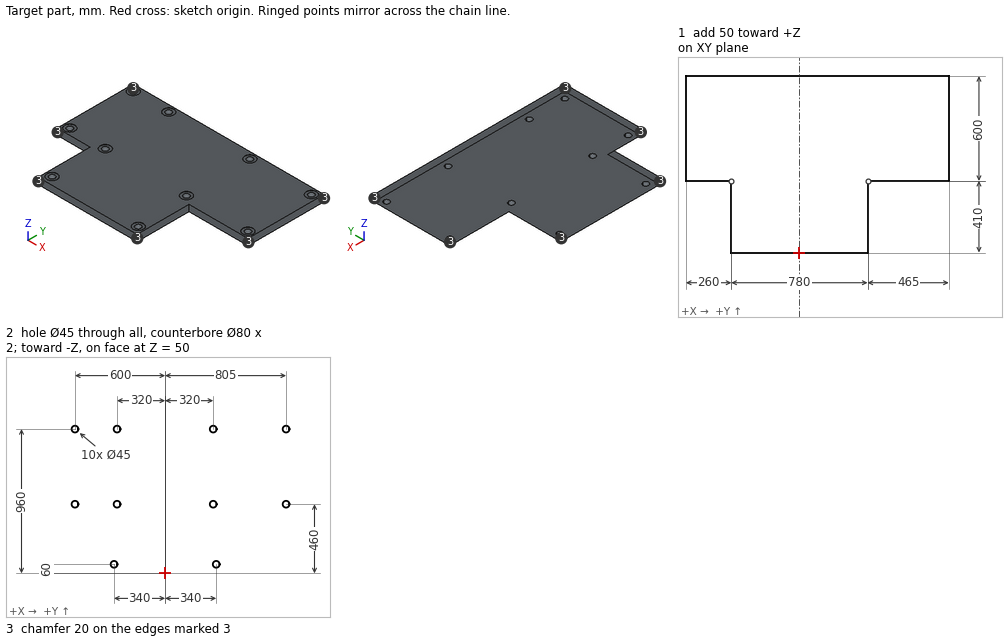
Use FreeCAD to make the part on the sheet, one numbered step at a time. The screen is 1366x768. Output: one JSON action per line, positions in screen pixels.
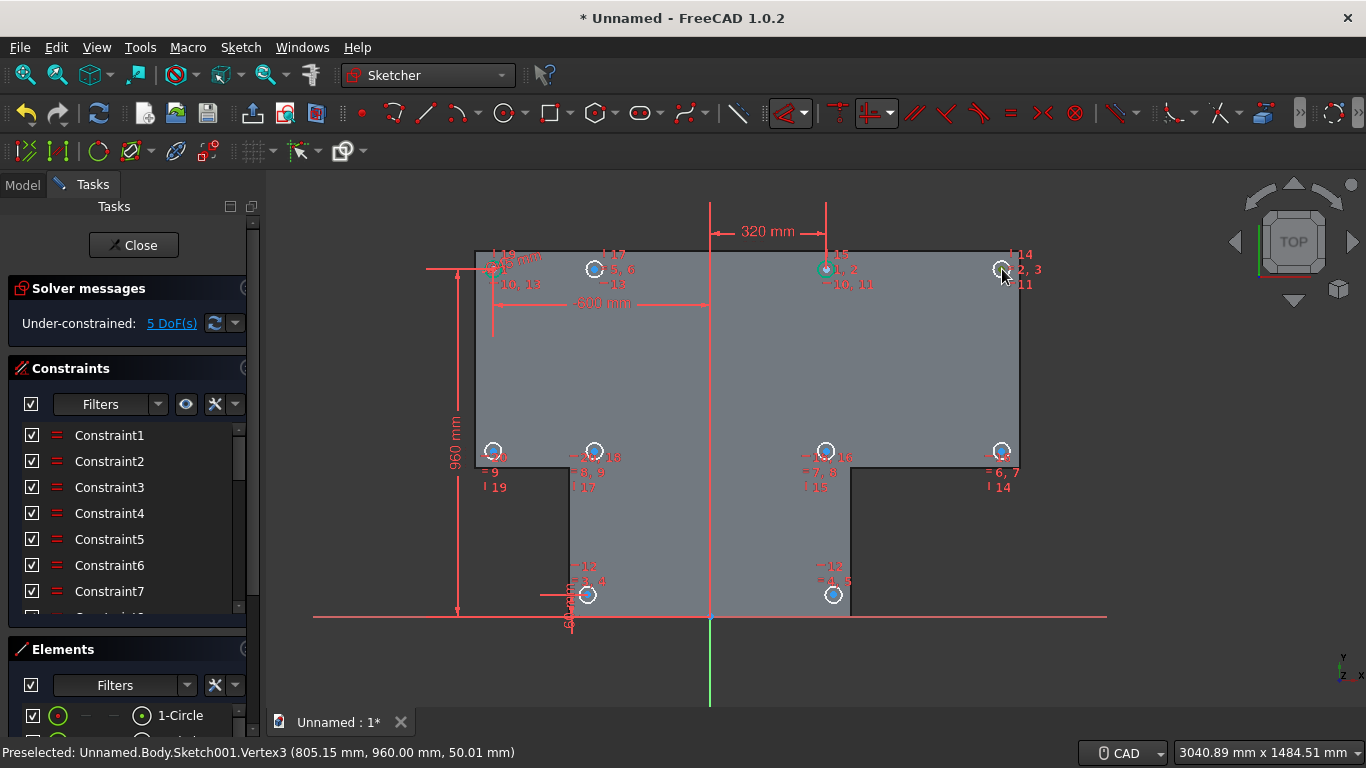
{"action": "key", "text": "l"}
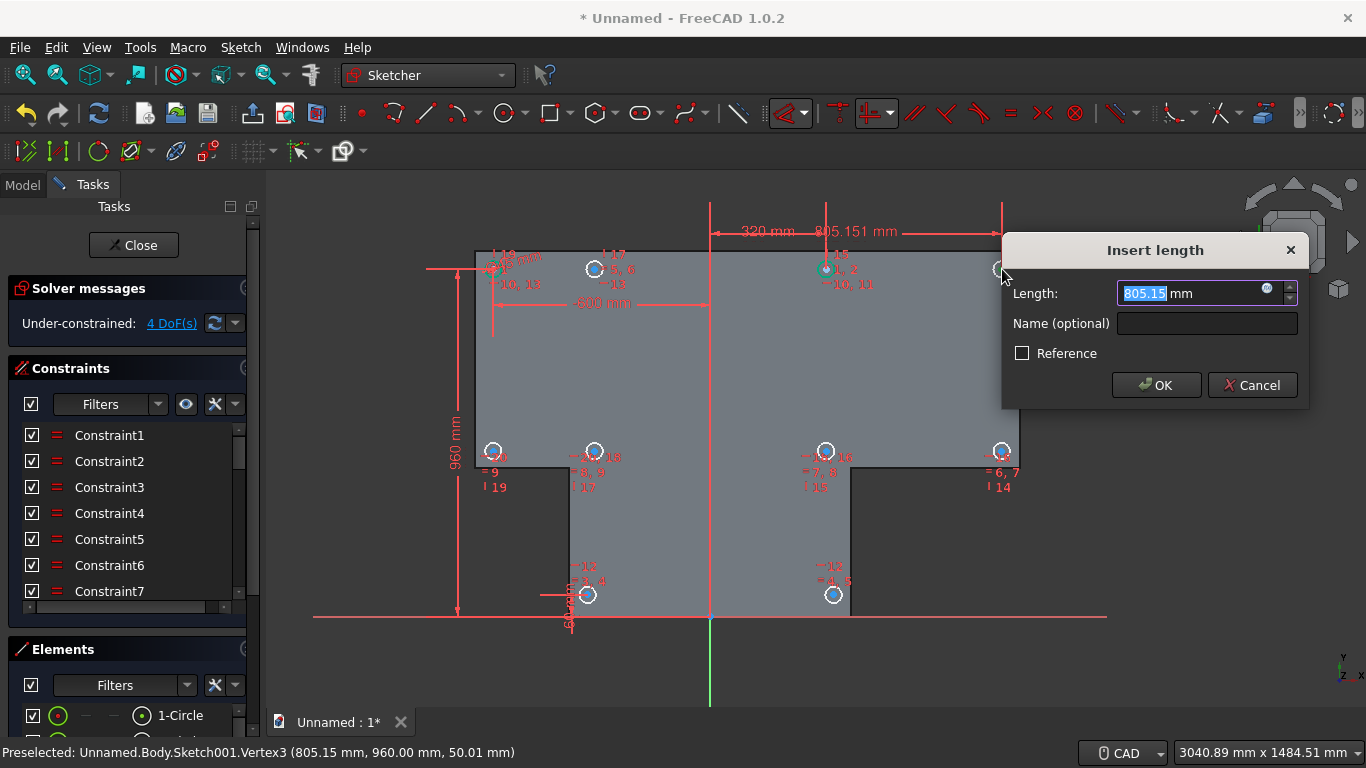
{"action": "type", "text": "805"}
{"action": "key", "text": "Return"}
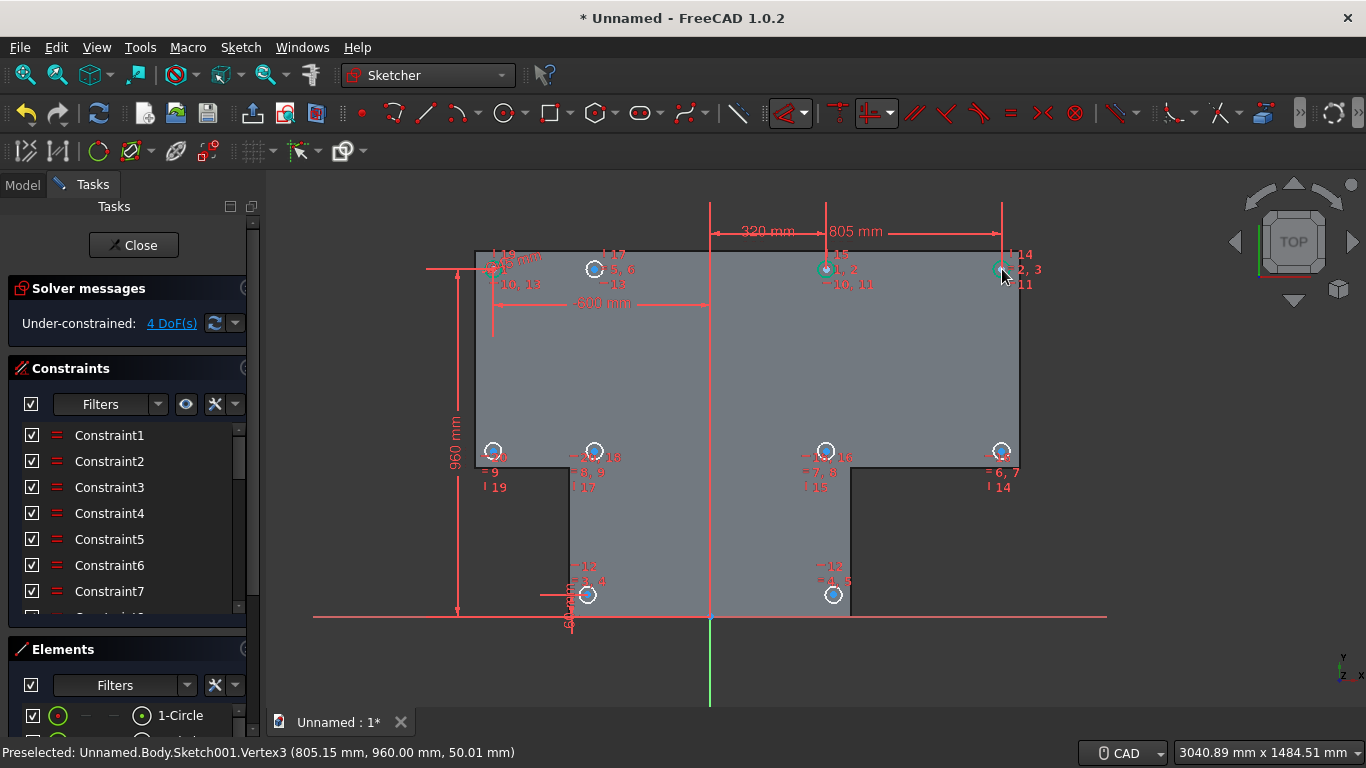
{"action": "left_click", "coordinate": [588, 595]}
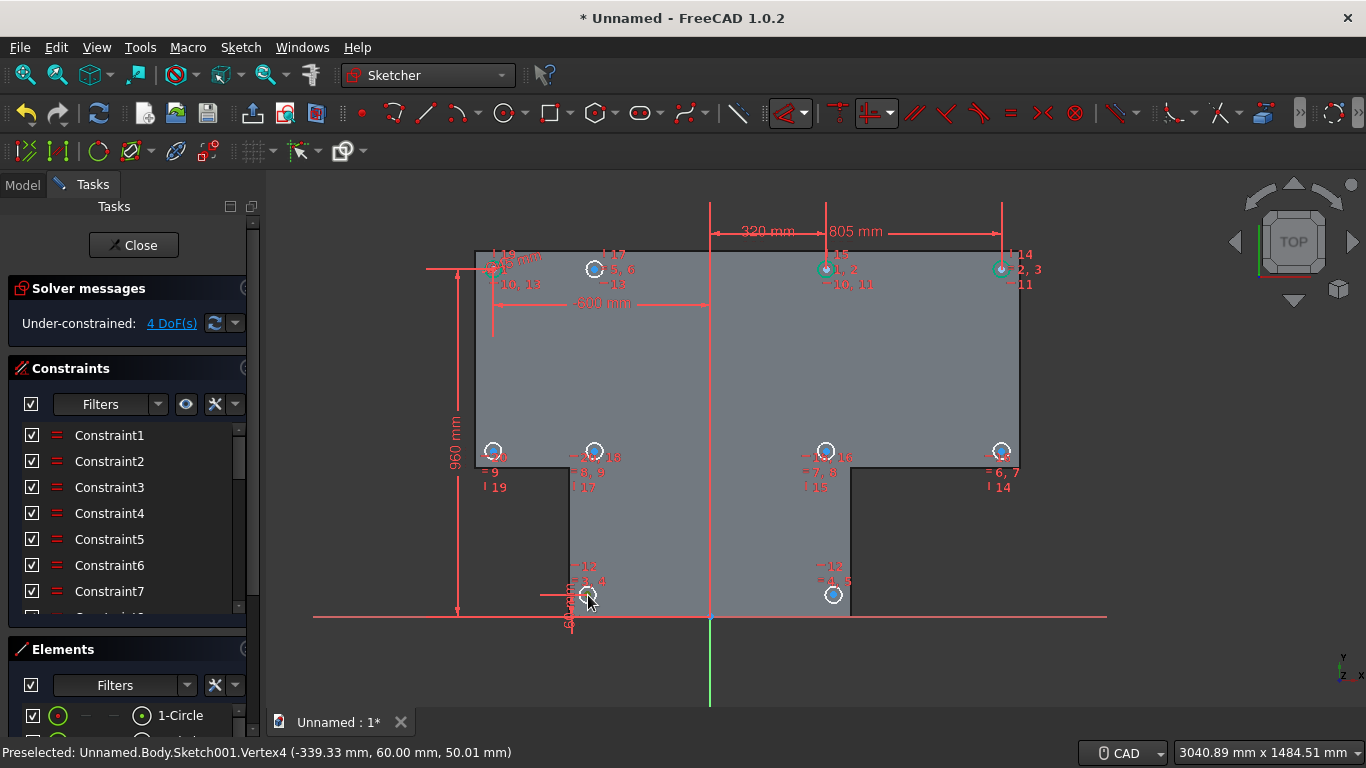
{"action": "left_click", "coordinate": [806, 114]}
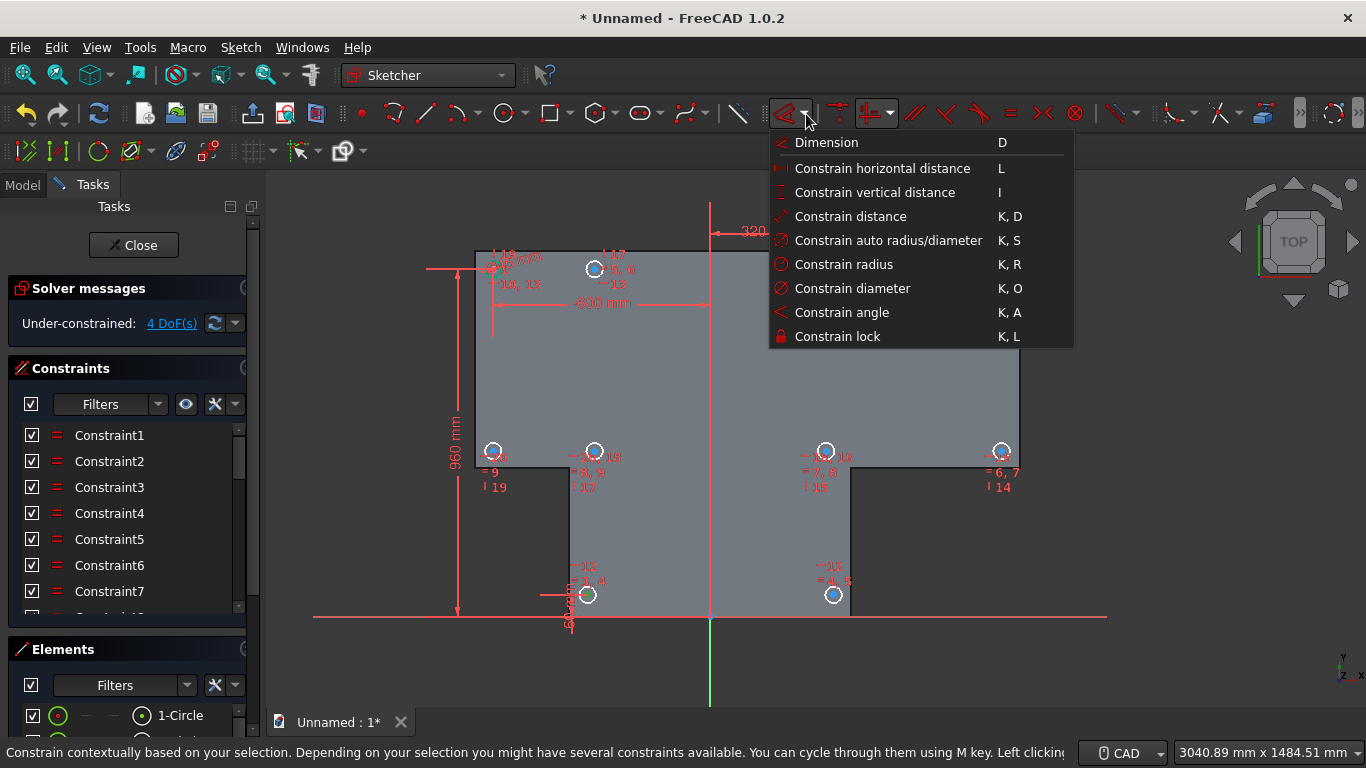
{"action": "left_click", "coordinate": [922, 168]}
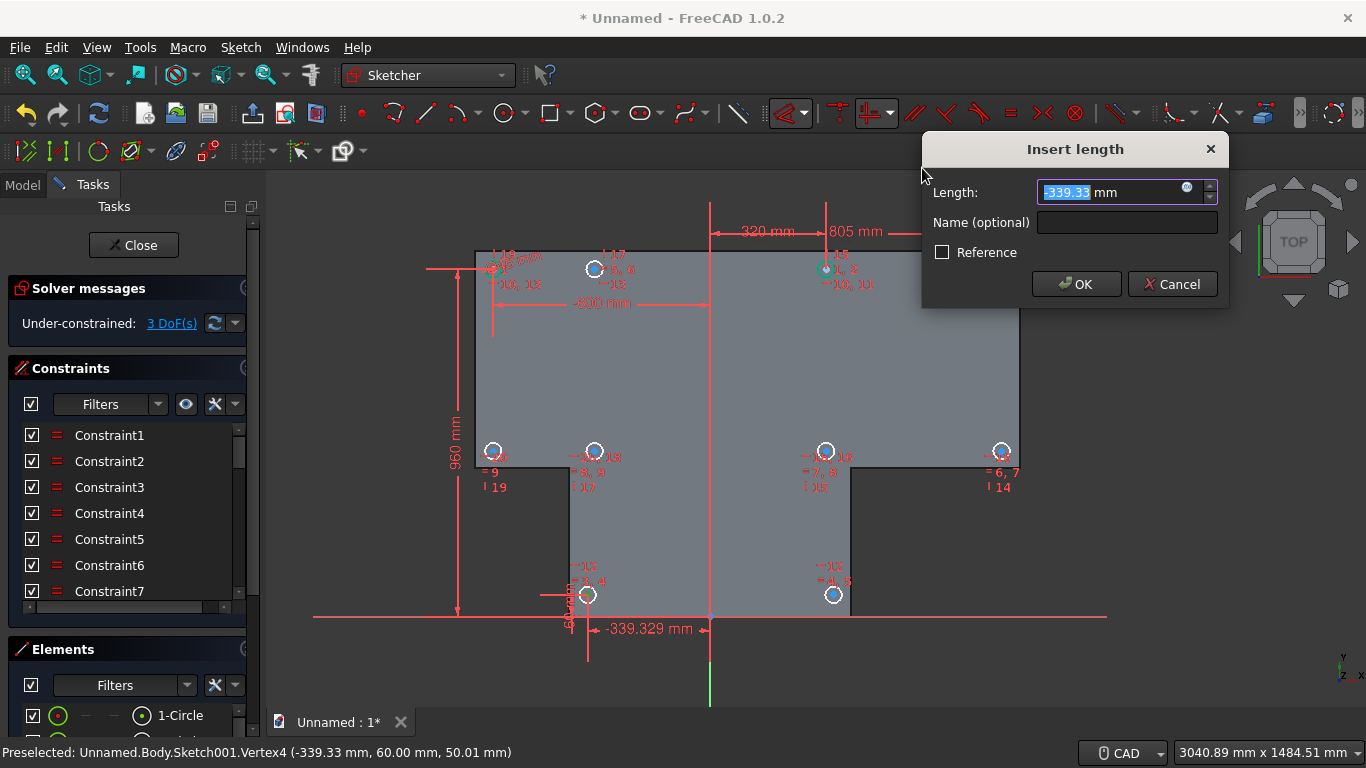
{"action": "type", "text": "-340"}
{"action": "key", "text": "Return"}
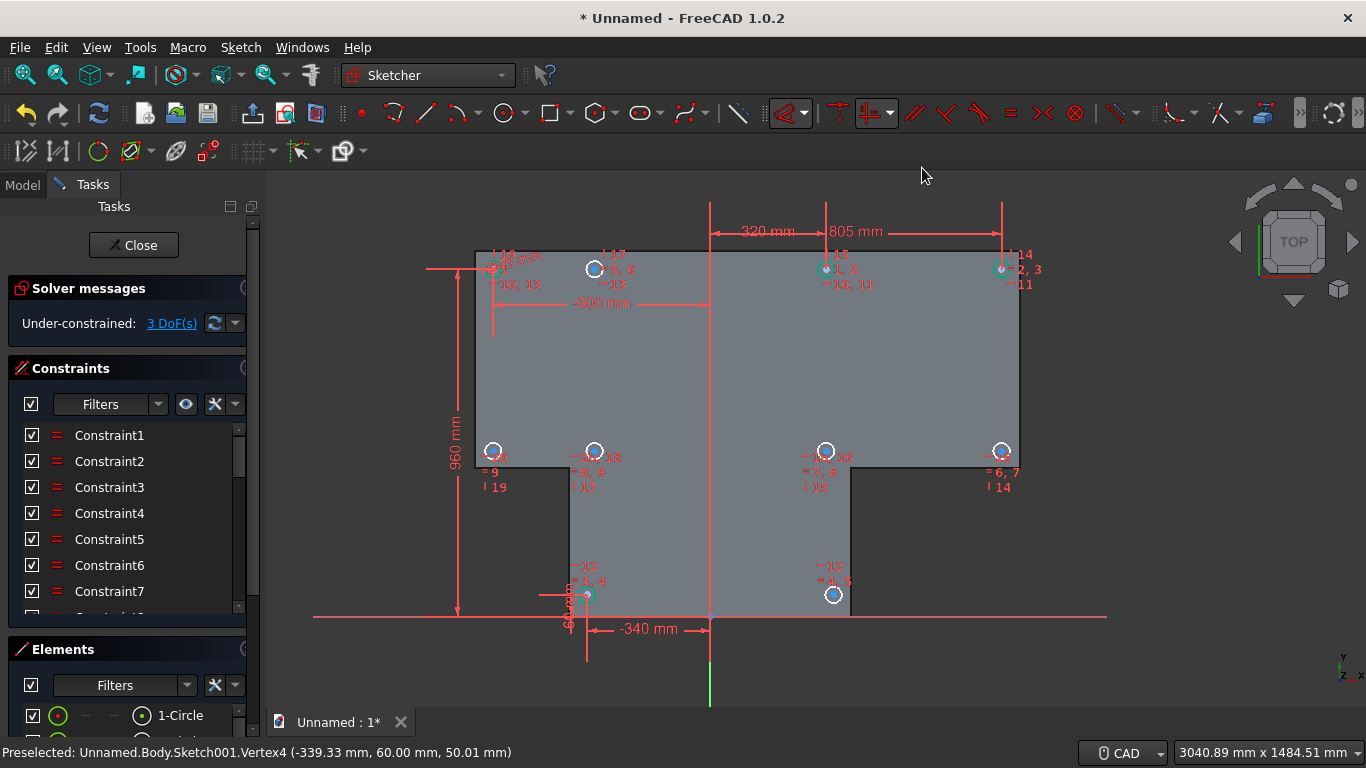
{"action": "left_click", "coordinate": [834, 595]}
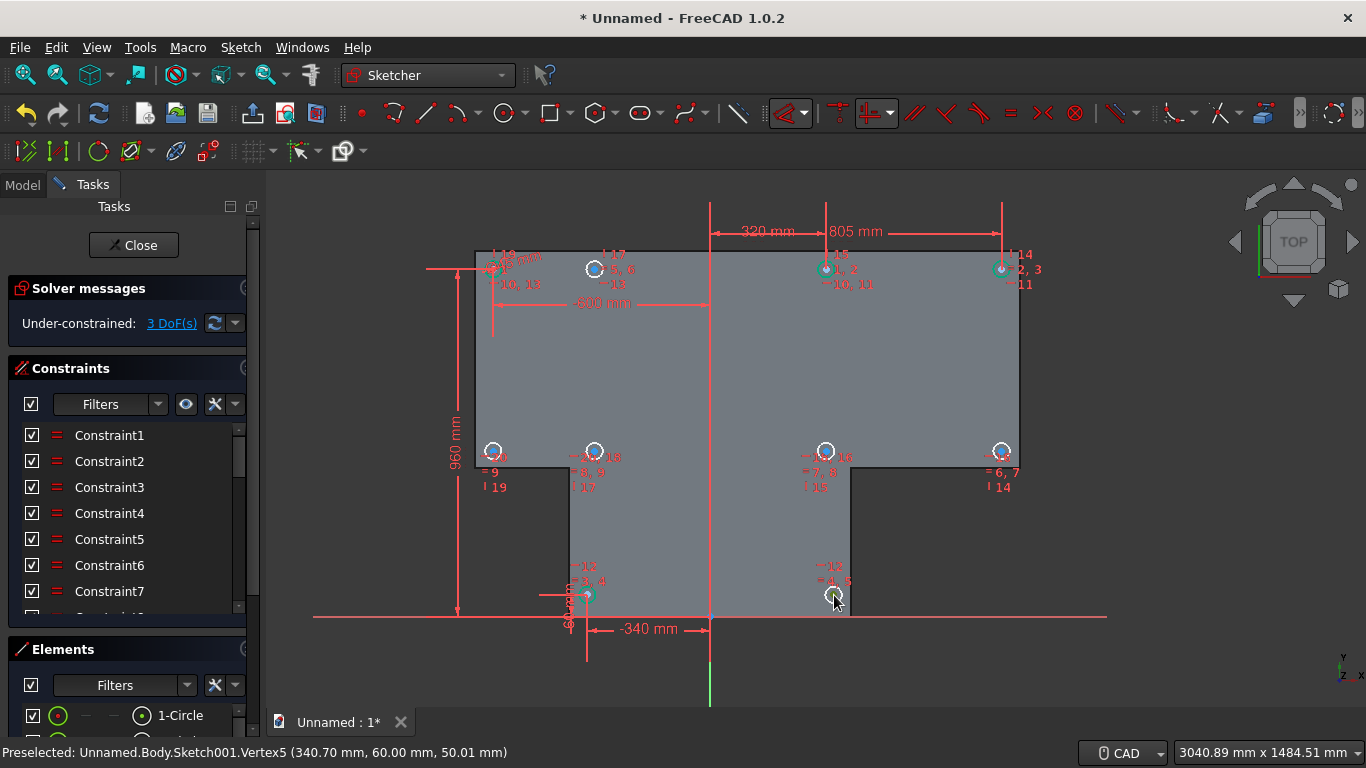
{"action": "left_click", "coordinate": [806, 114]}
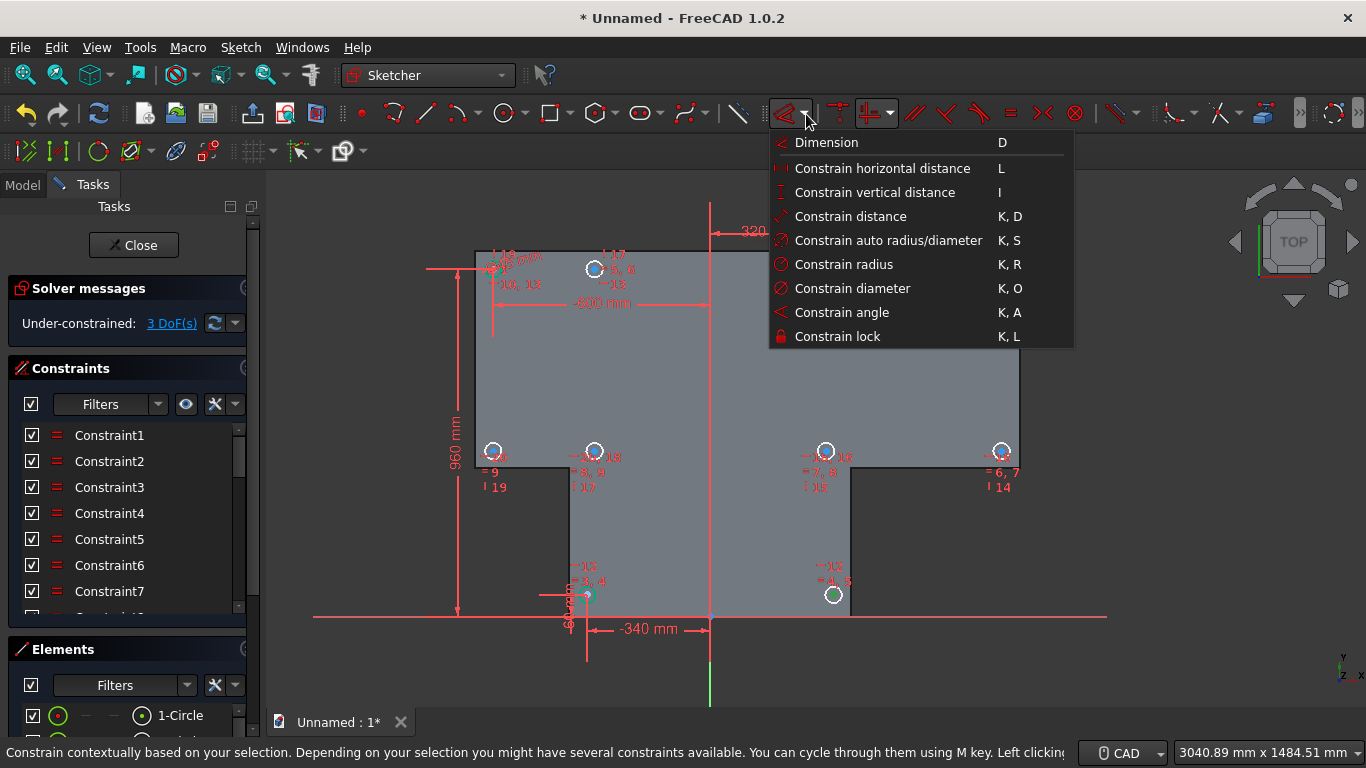
{"action": "left_click", "coordinate": [922, 168]}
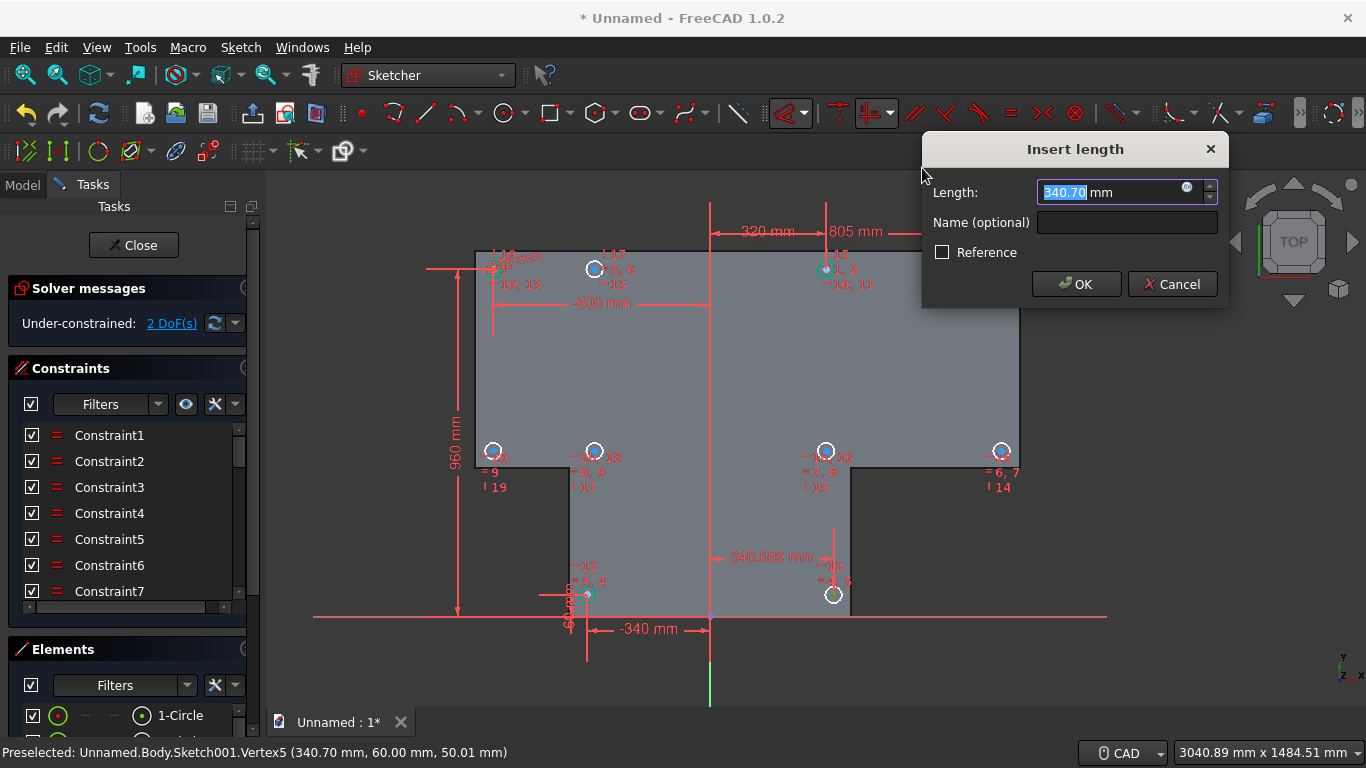
{"action": "type", "text": "340"}
{"action": "key", "text": "Return"}